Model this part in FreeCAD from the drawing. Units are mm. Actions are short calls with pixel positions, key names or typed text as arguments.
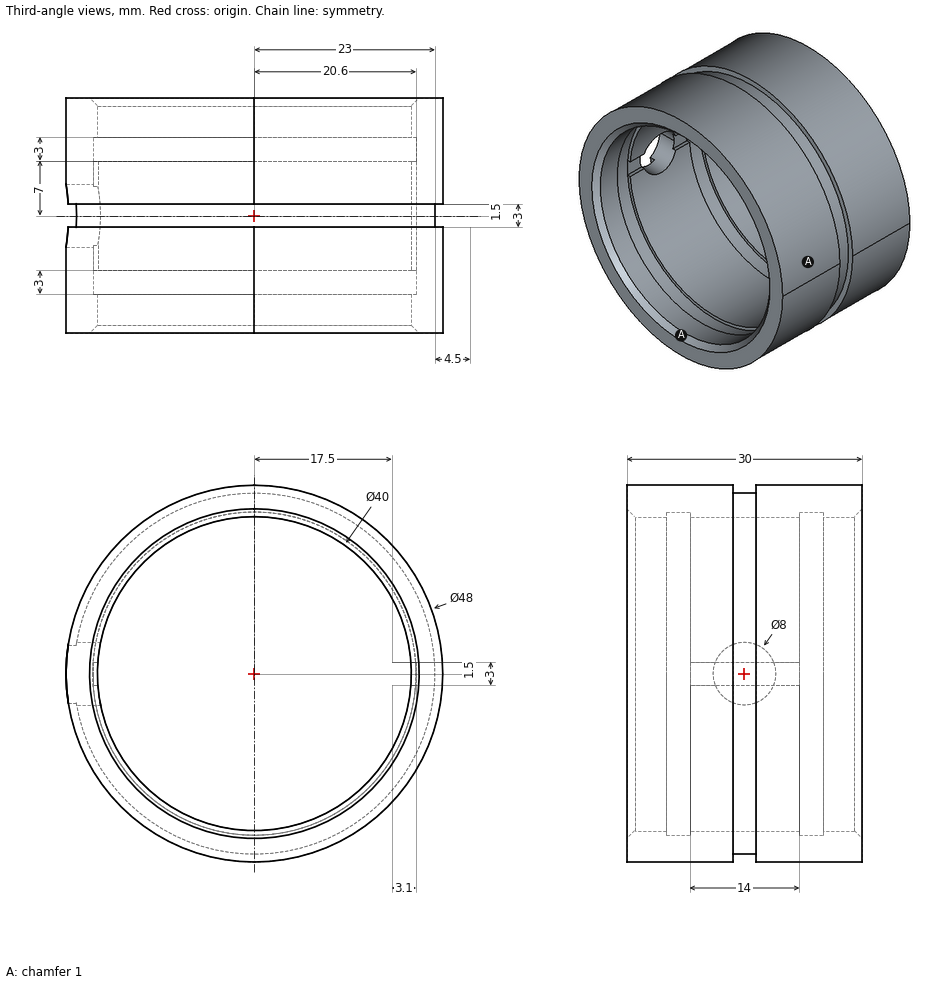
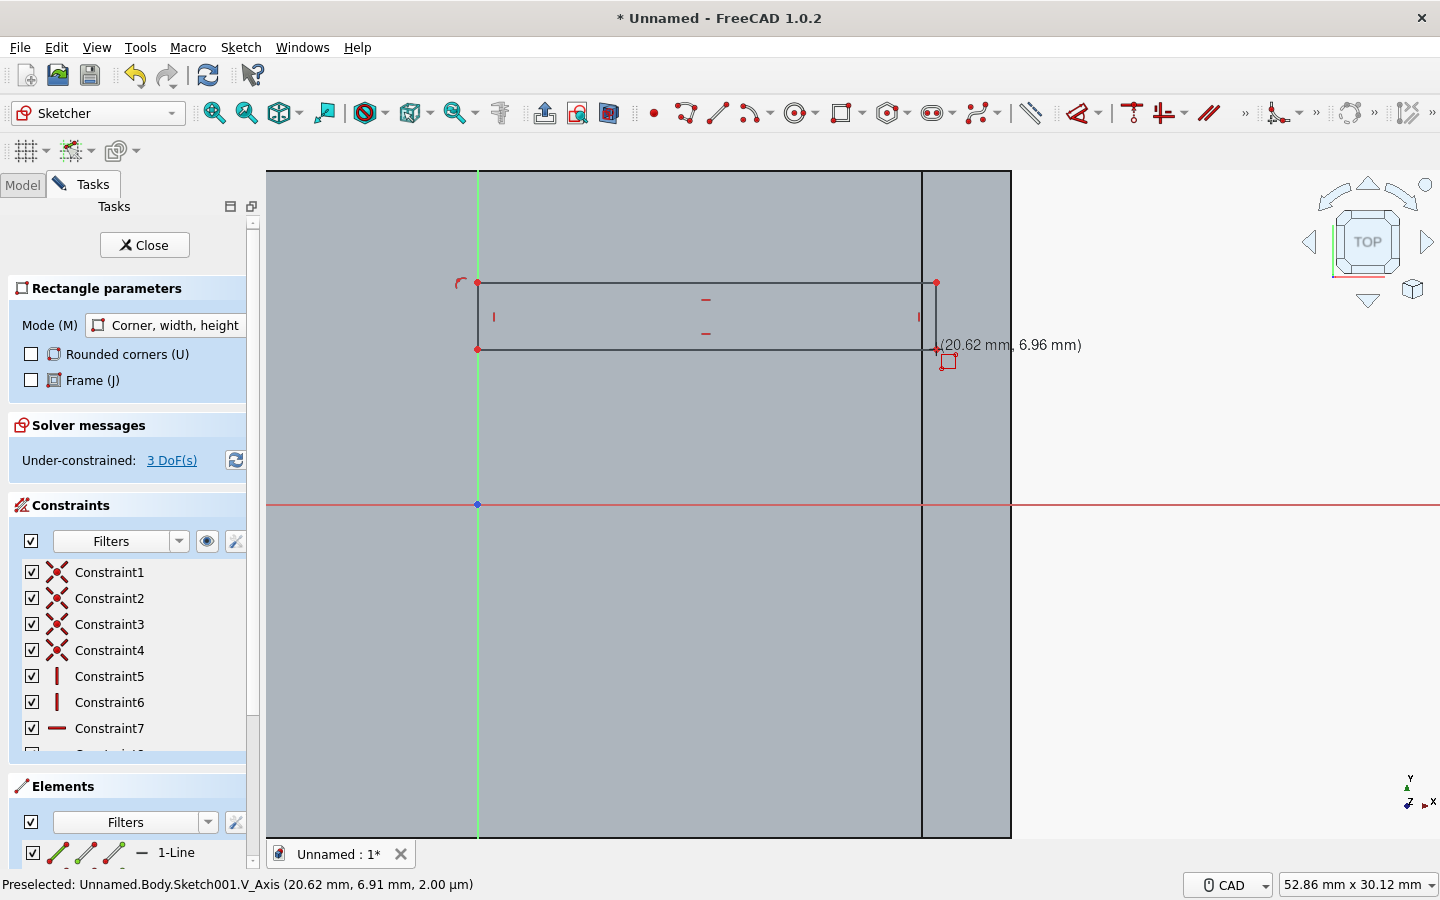
click(478, 660)
click(936, 727)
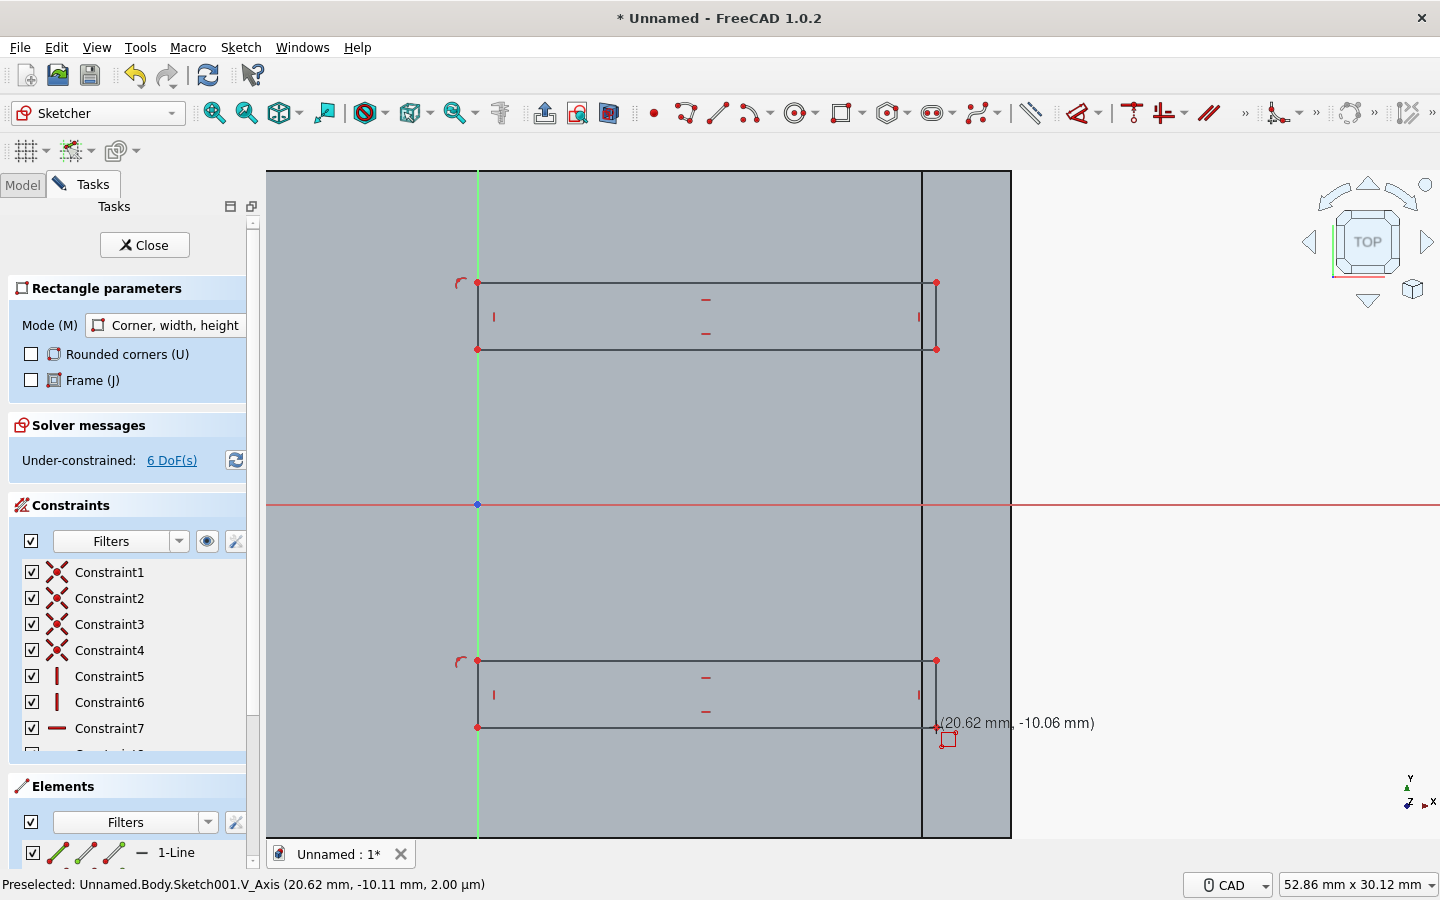
click(989, 471)
click(1089, 538)
key(Escape)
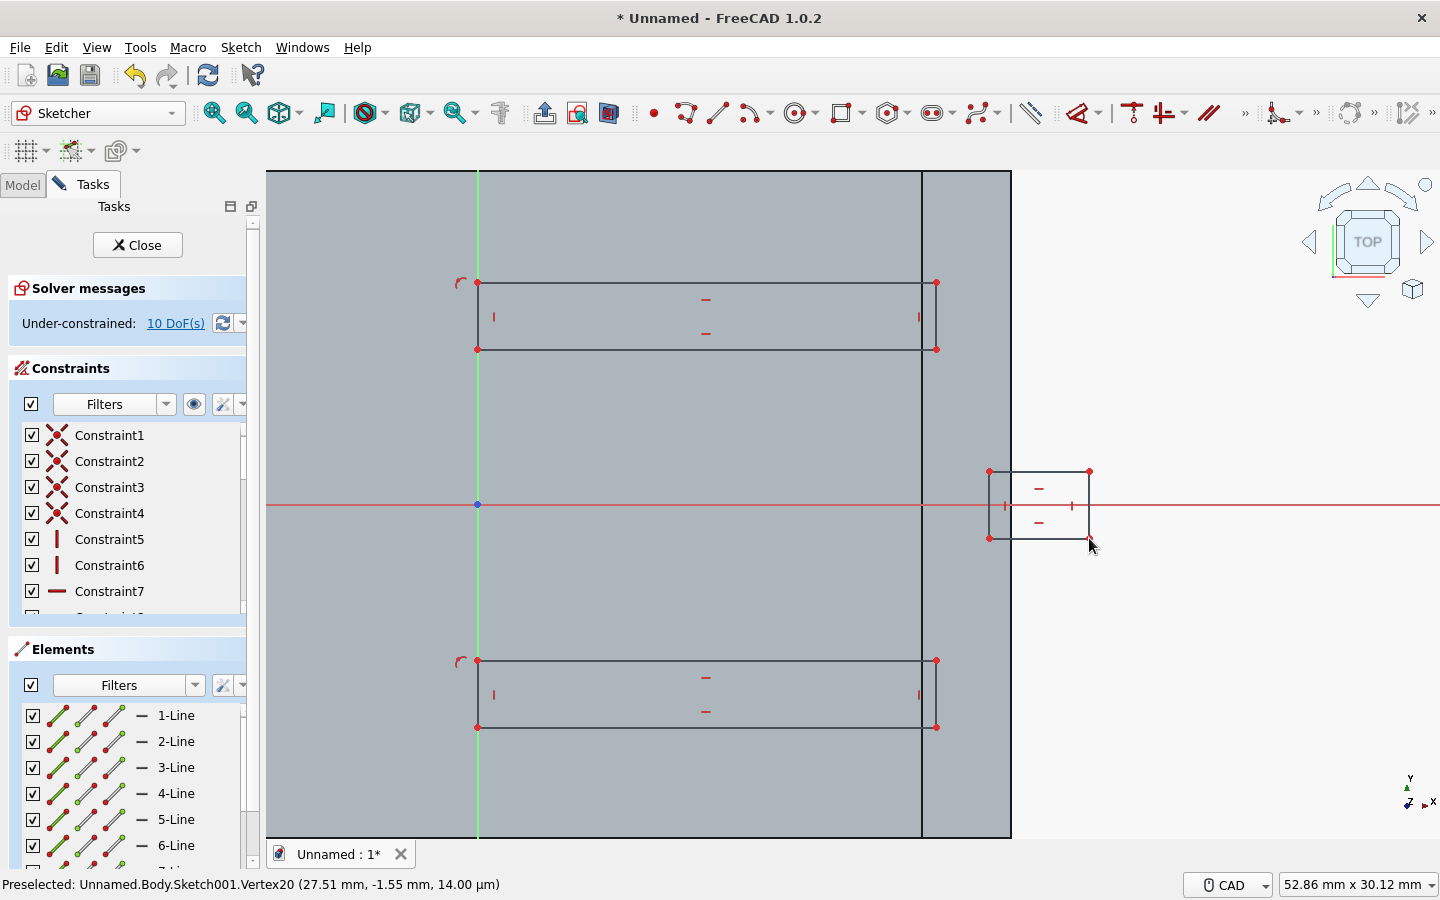
click(936, 283)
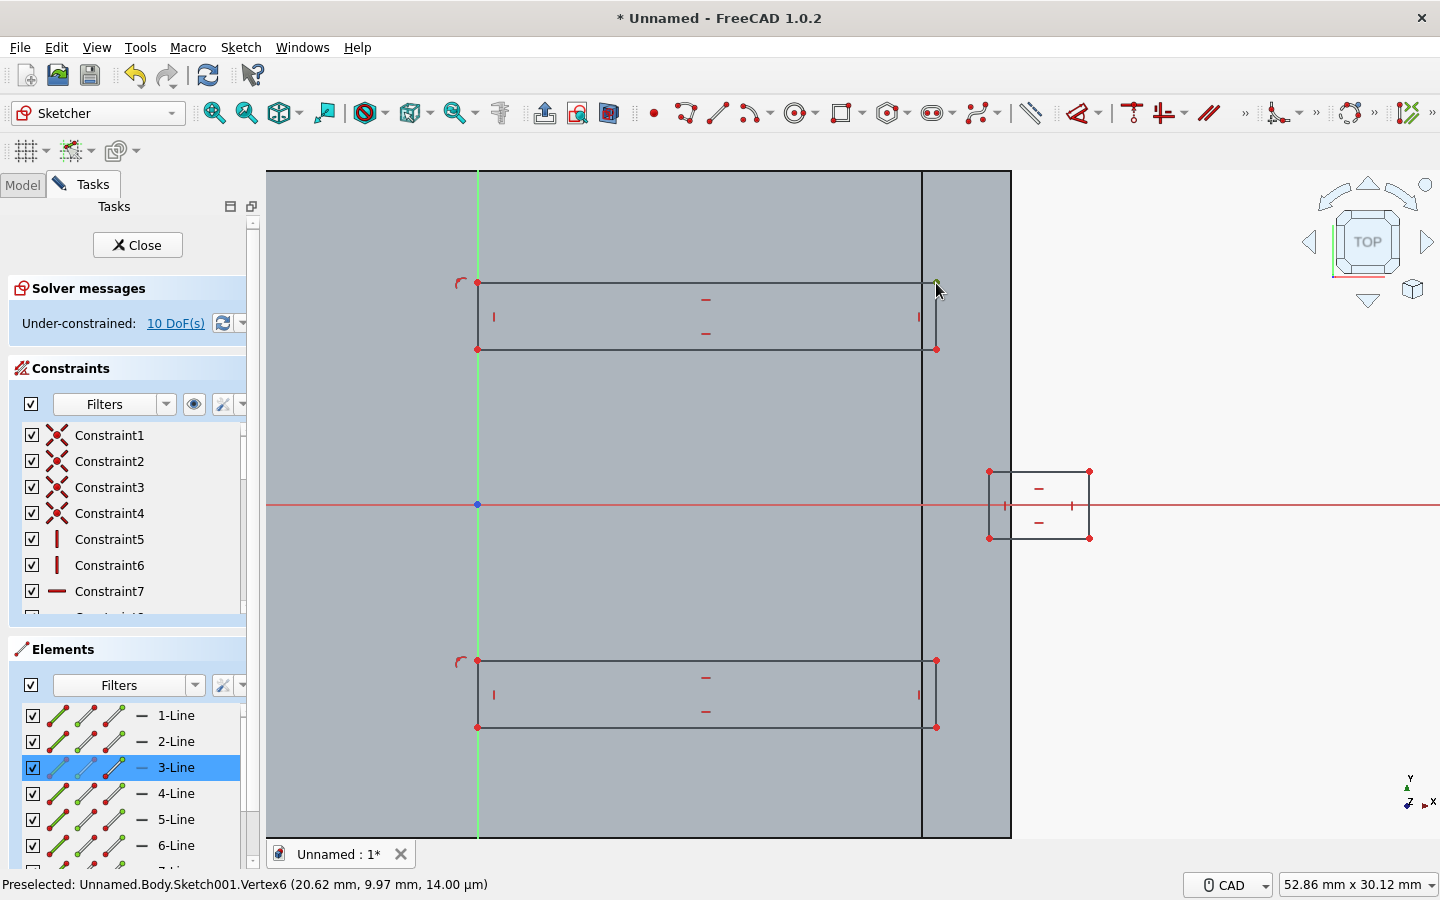
click(936, 728)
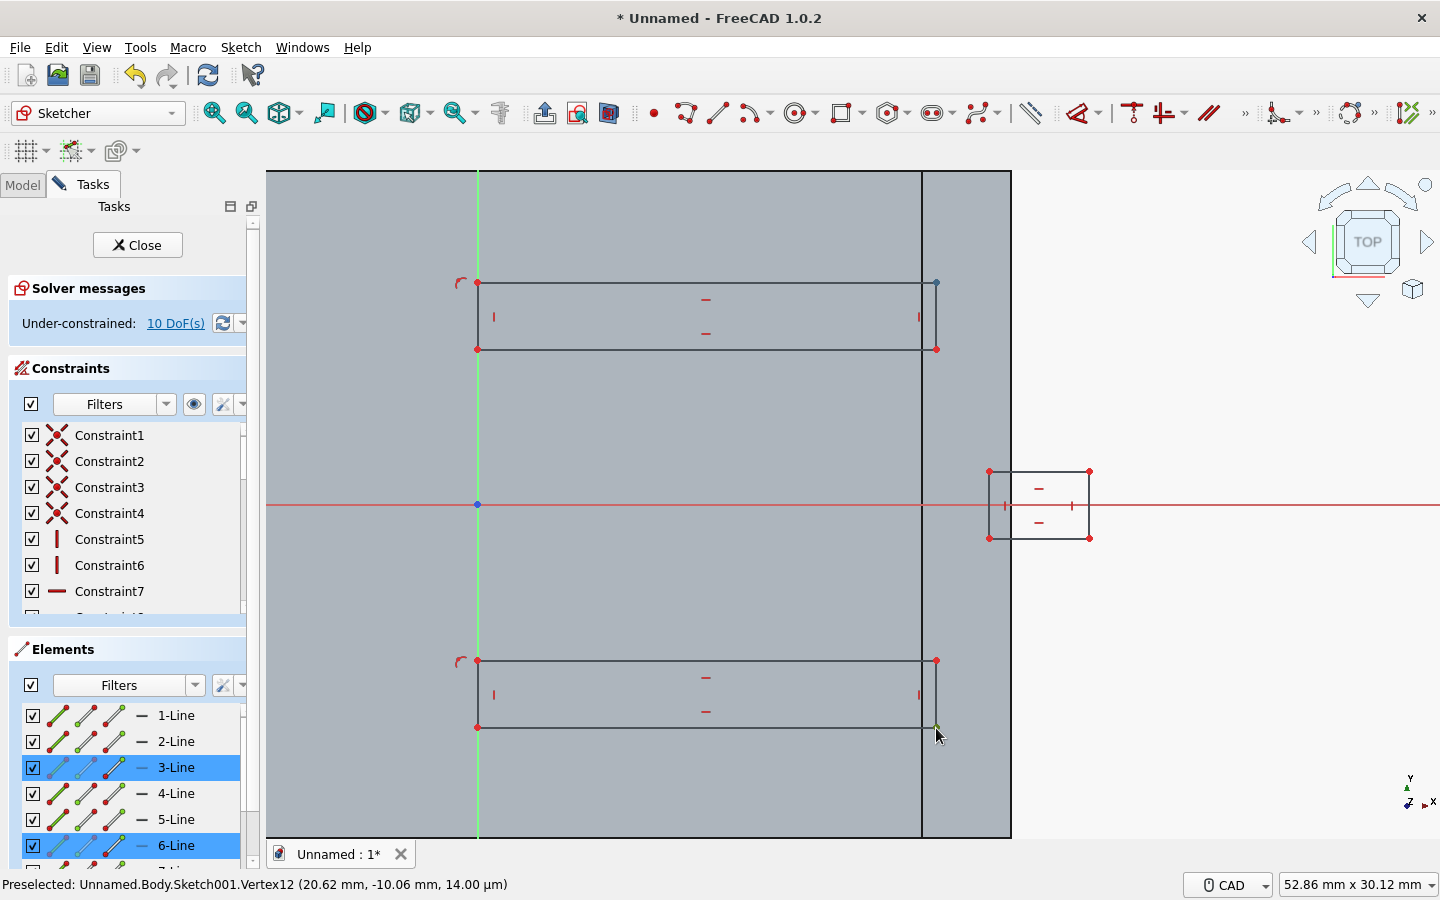
click(364, 504)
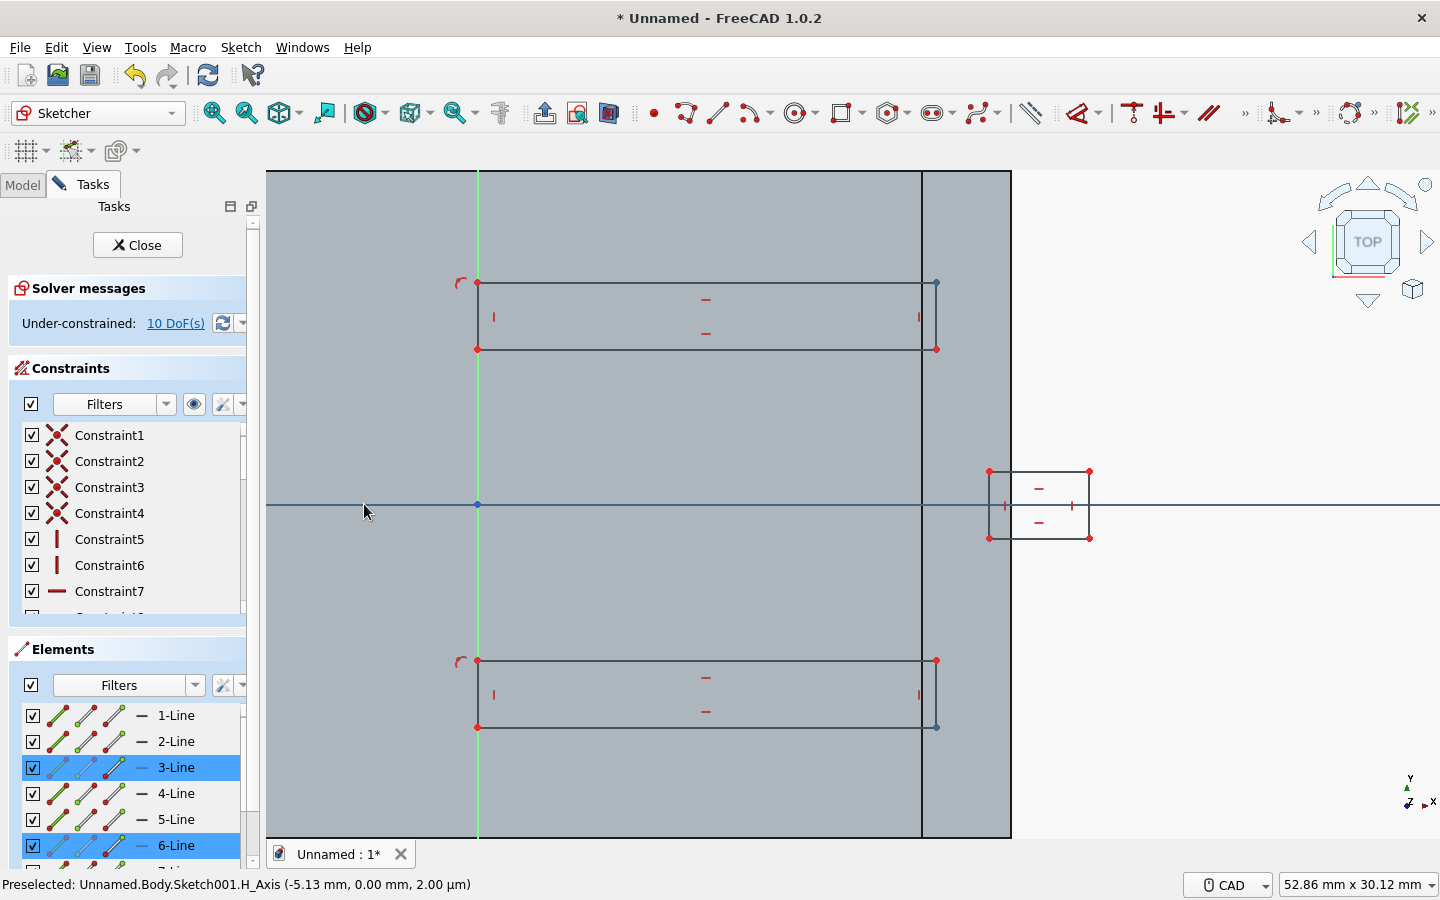
key(s)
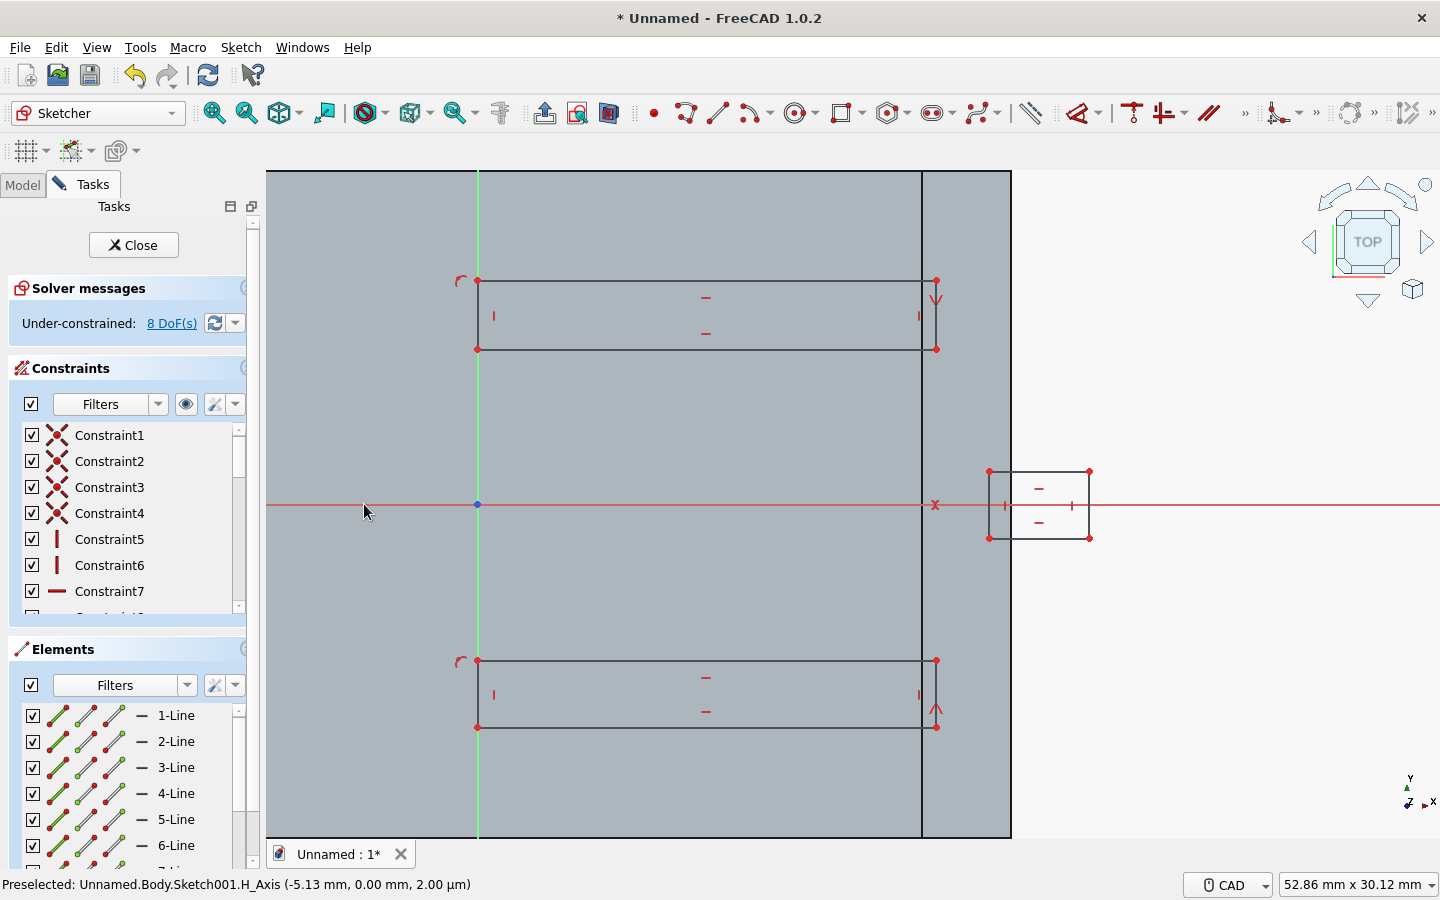
click(1078, 114)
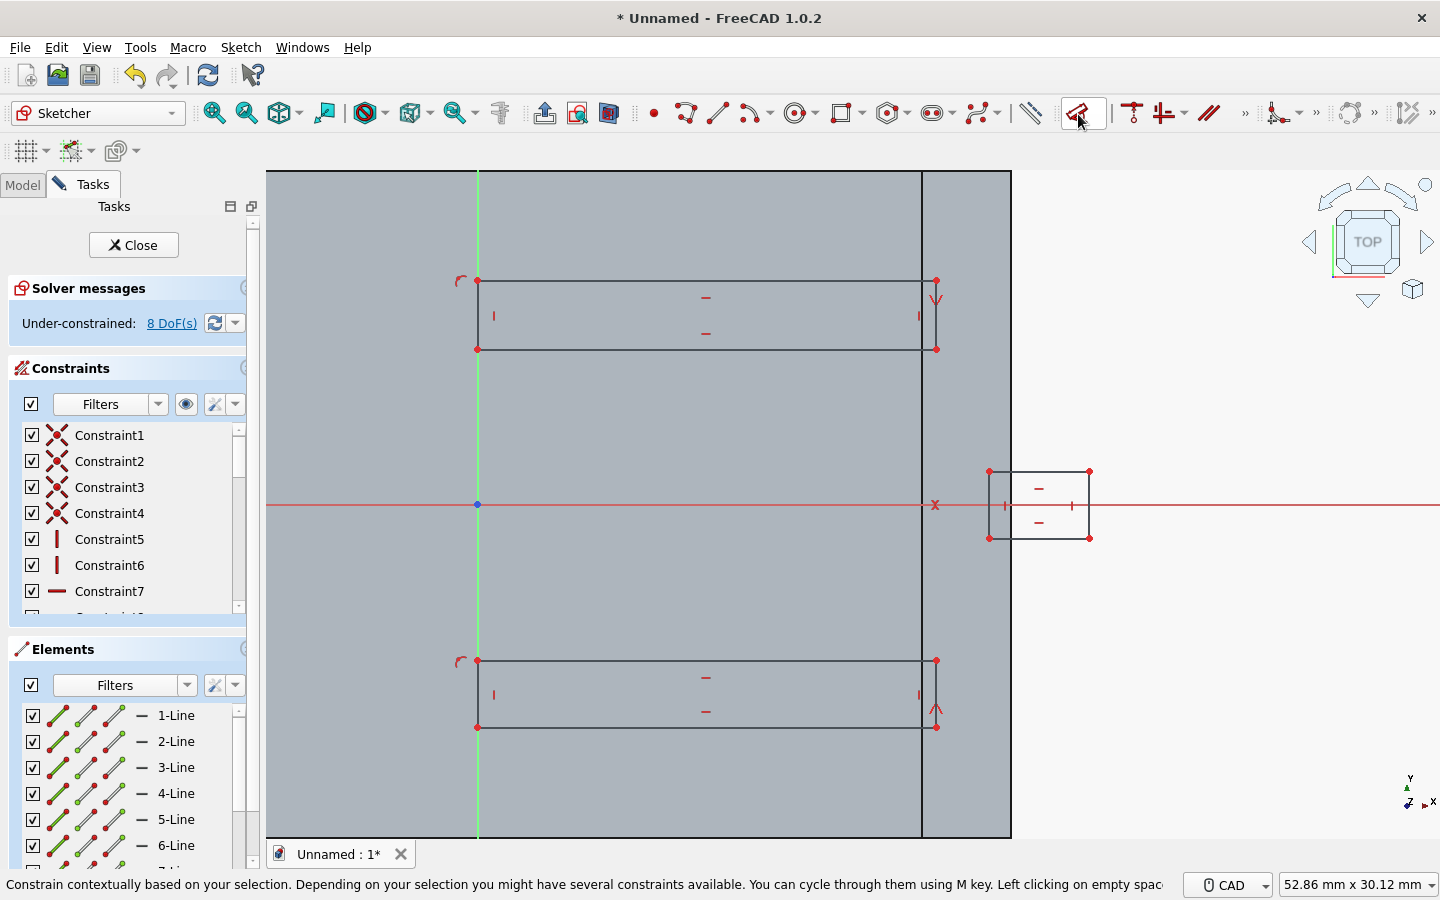
click(478, 302)
click(444, 315)